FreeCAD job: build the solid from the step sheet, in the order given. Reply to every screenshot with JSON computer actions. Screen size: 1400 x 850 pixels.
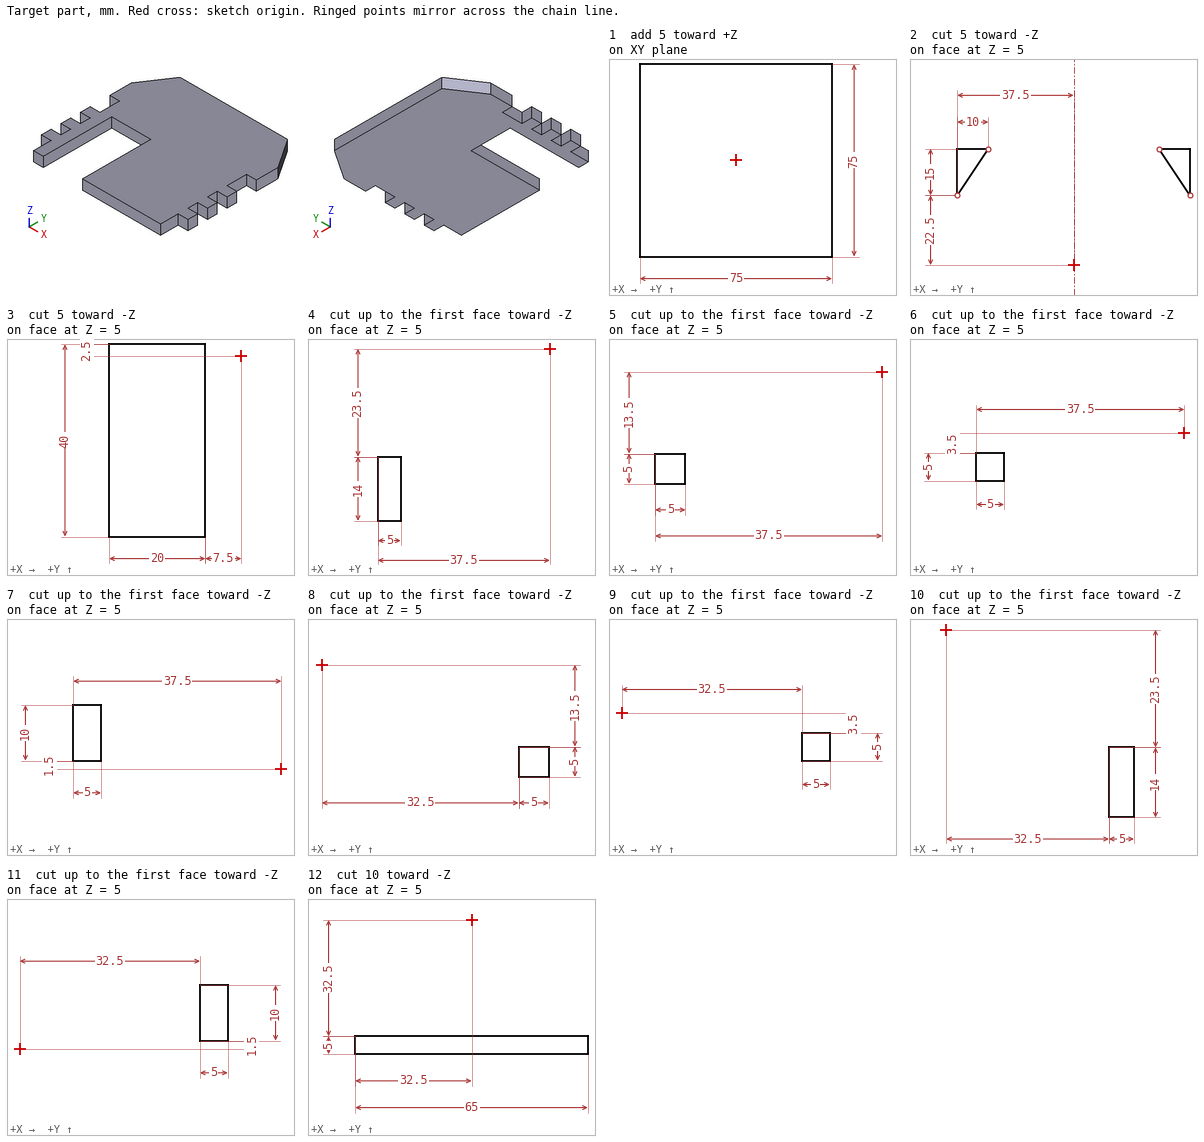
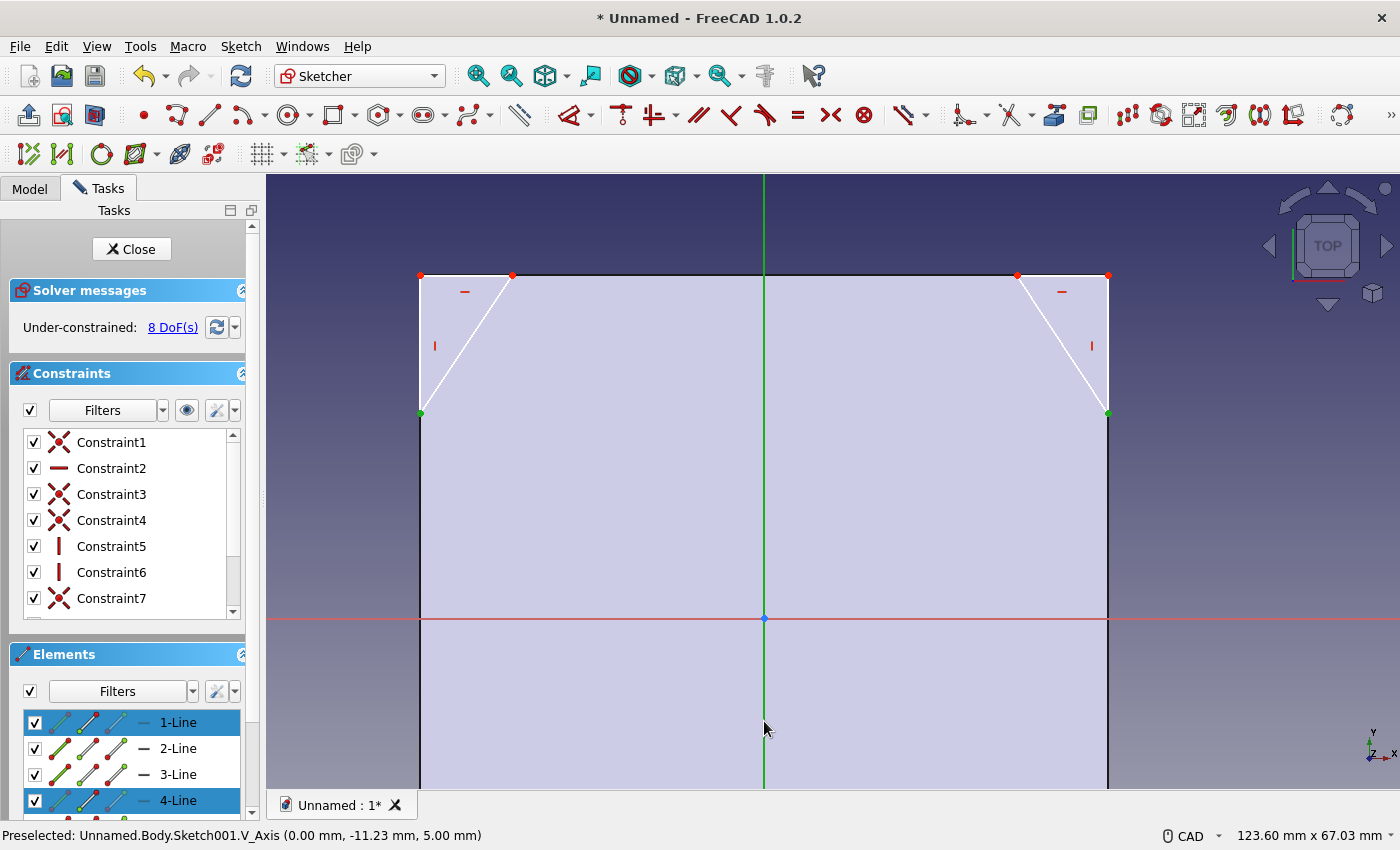
{"action": "left_click", "coordinate": [831, 116]}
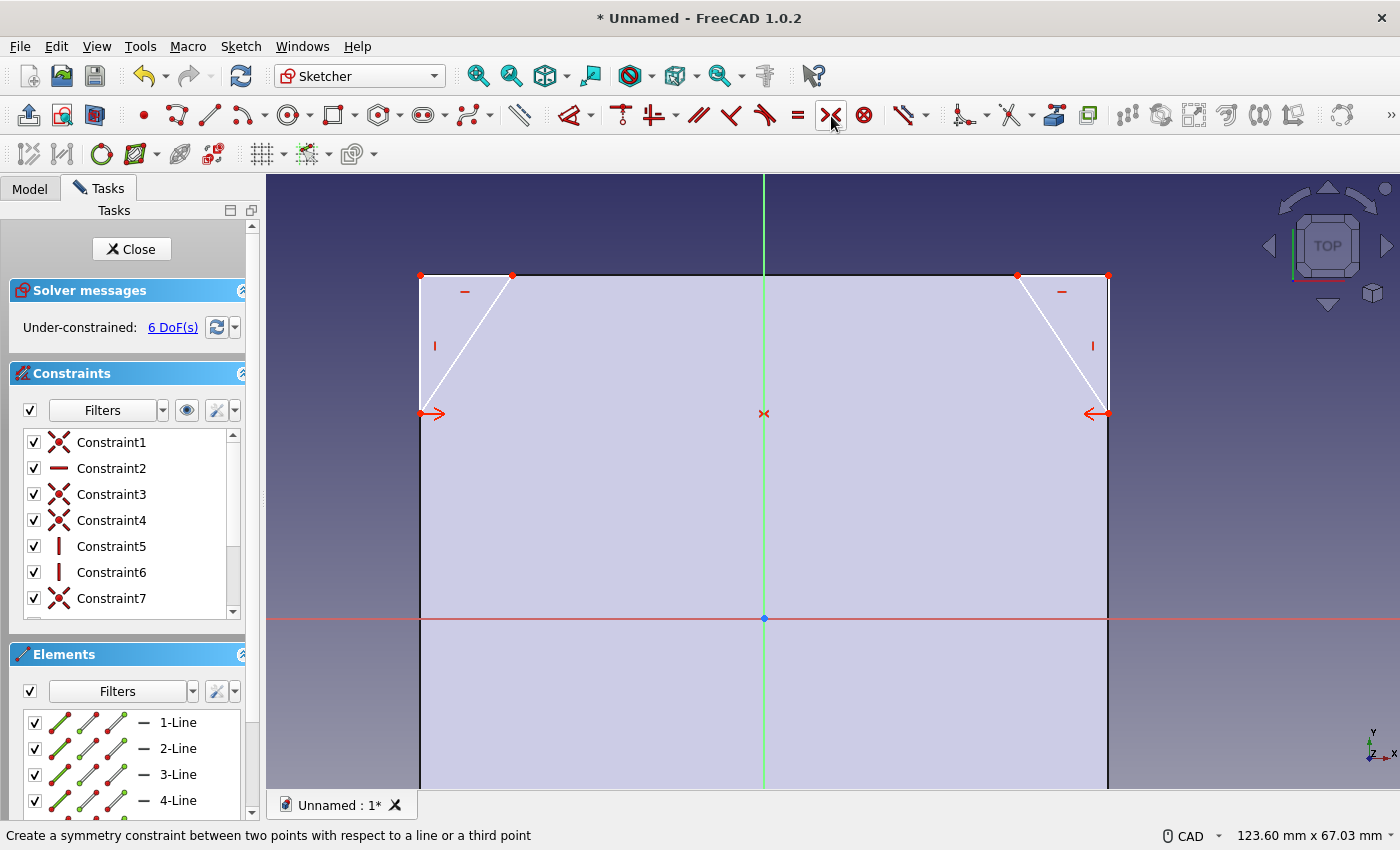
{"action": "left_click", "coordinate": [512, 276]}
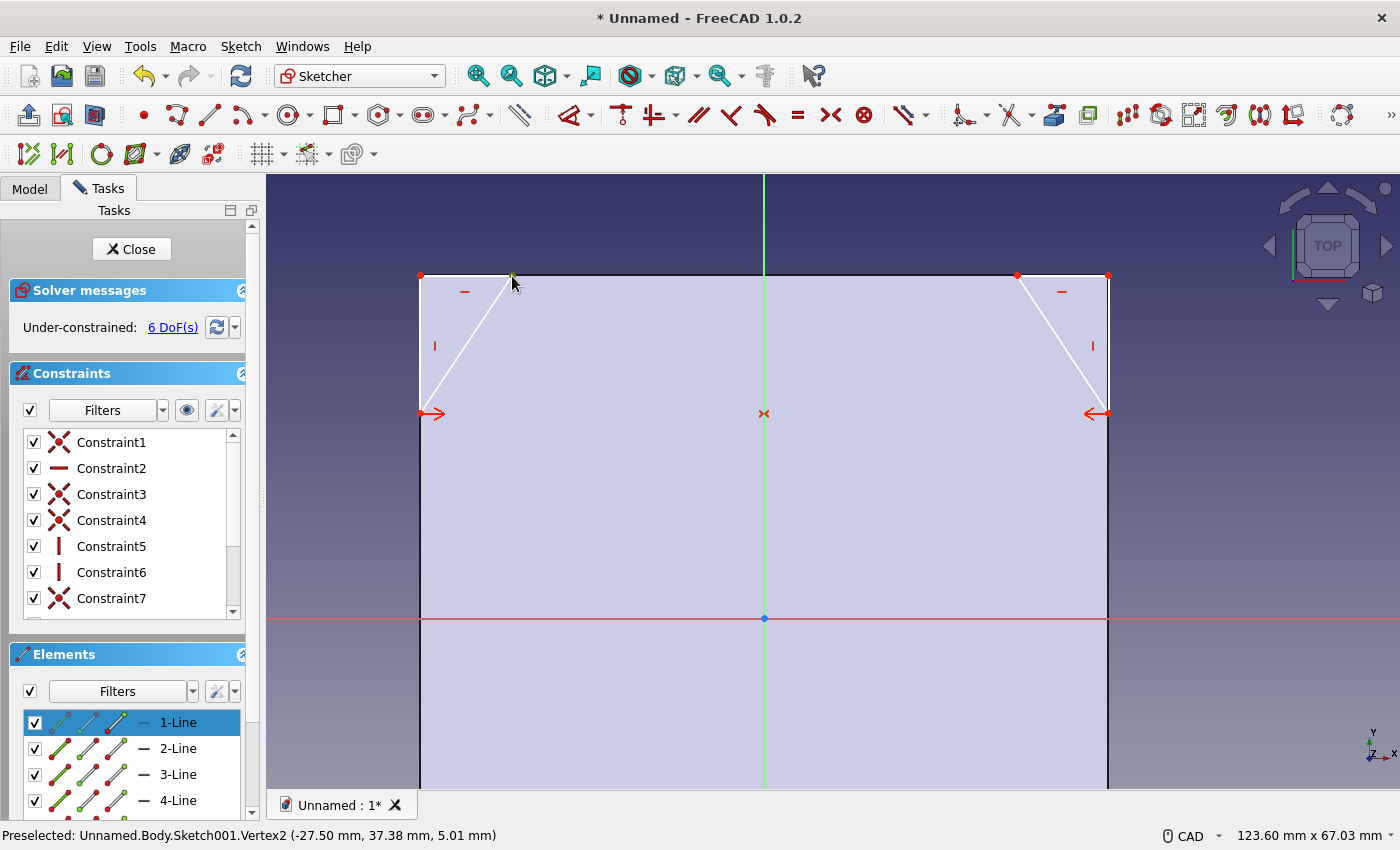
{"action": "left_click", "coordinate": [1017, 276]}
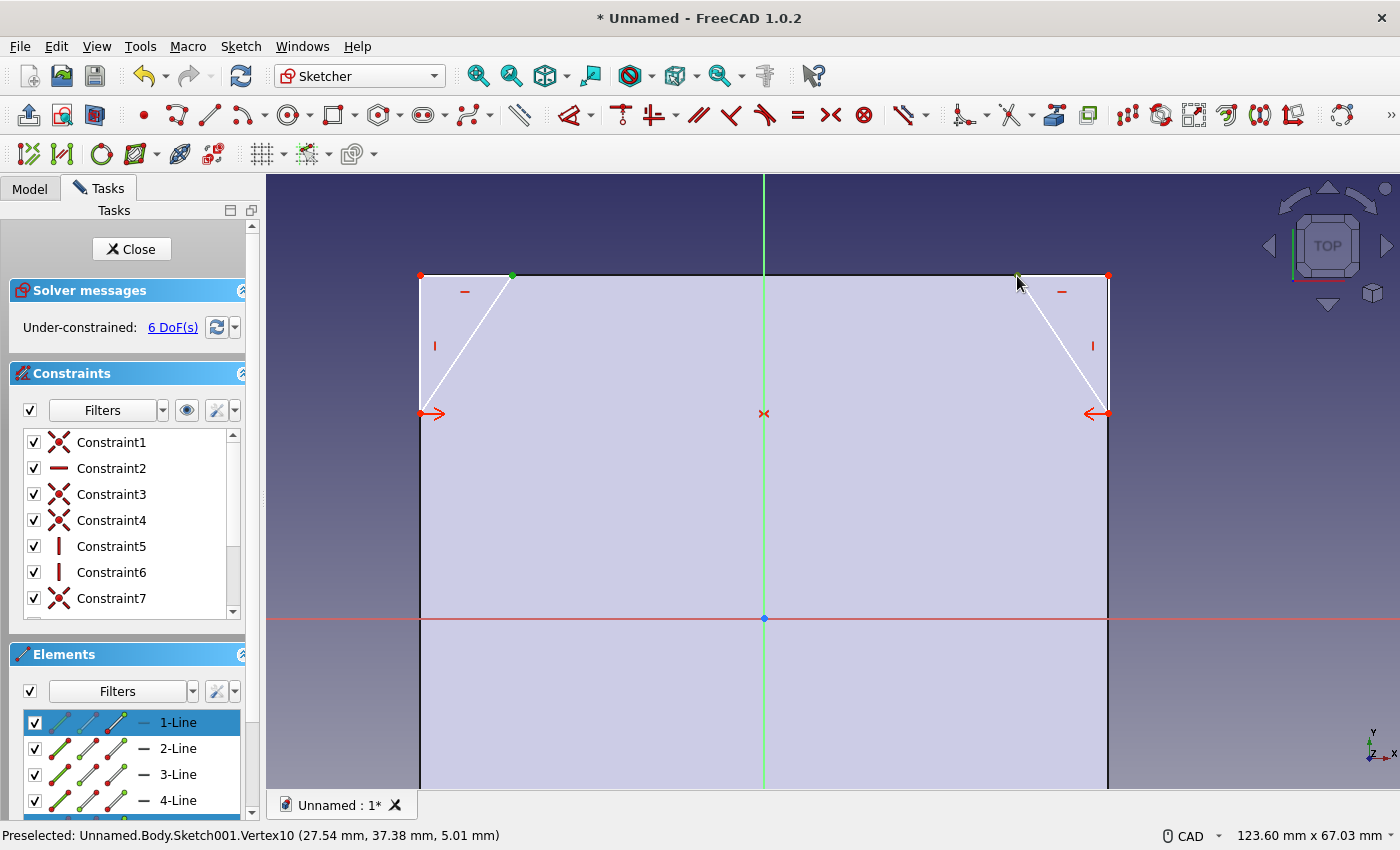
{"action": "left_click", "coordinate": [764, 721]}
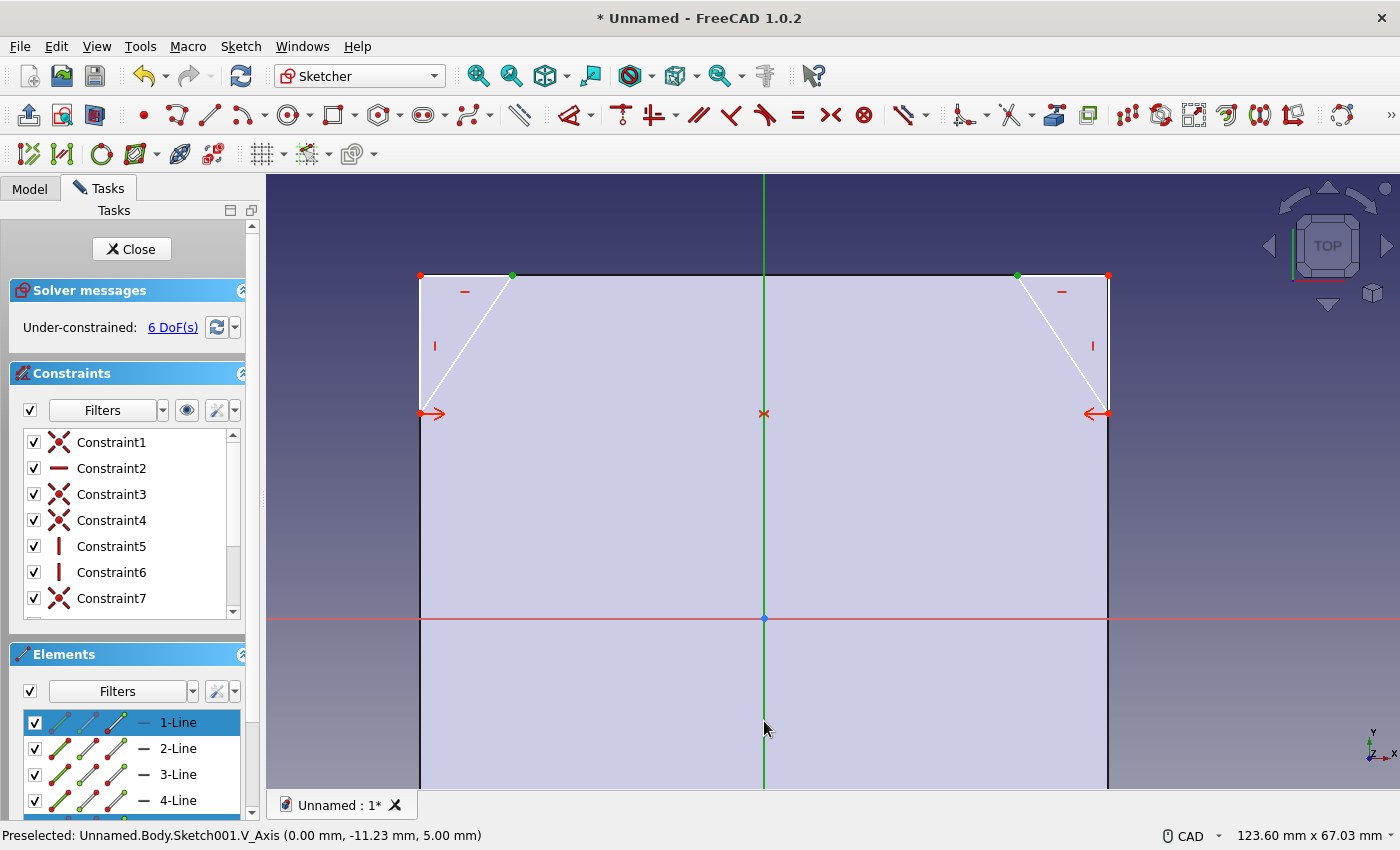
{"action": "left_click", "coordinate": [831, 116]}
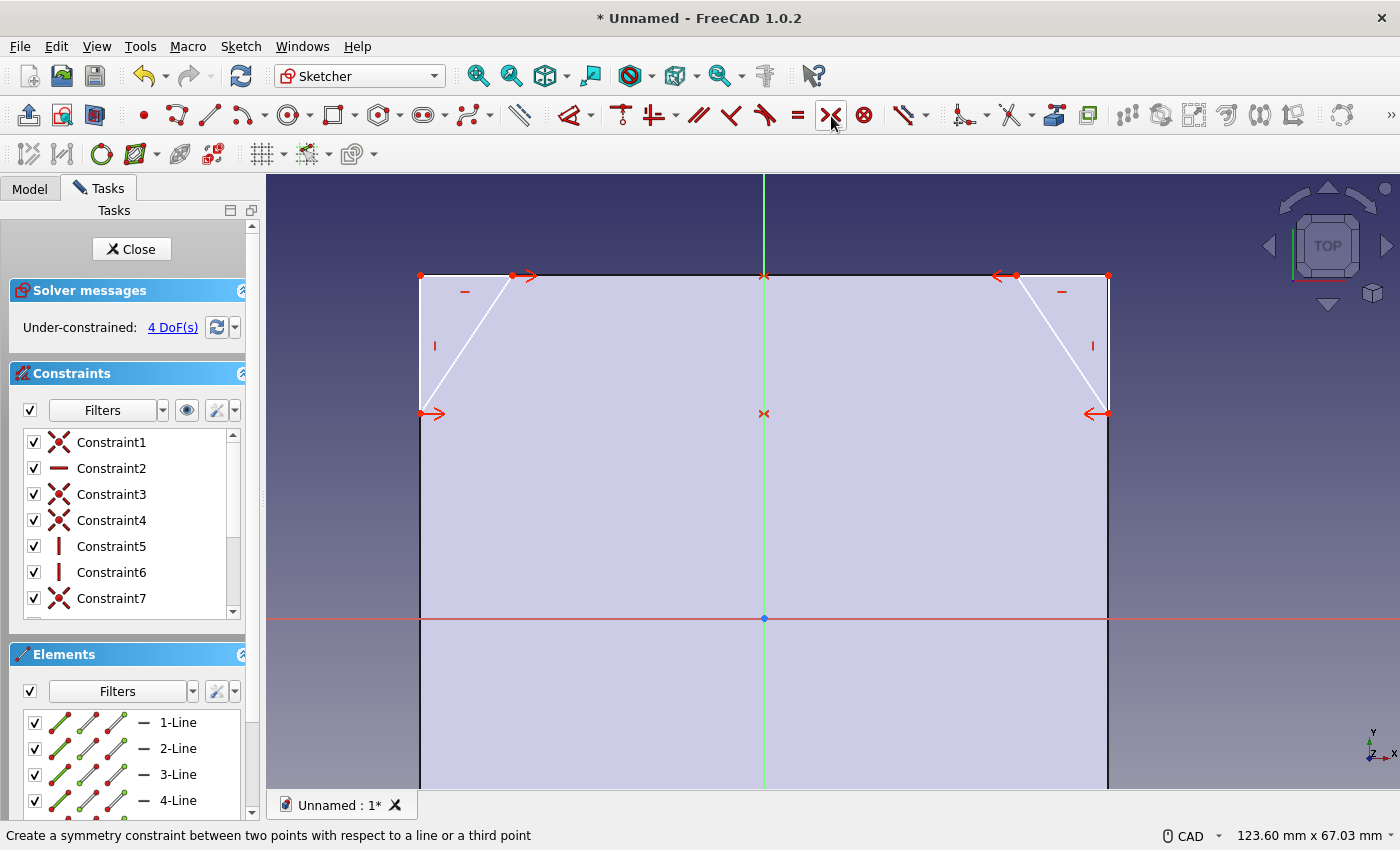
{"action": "left_click", "coordinate": [568, 116]}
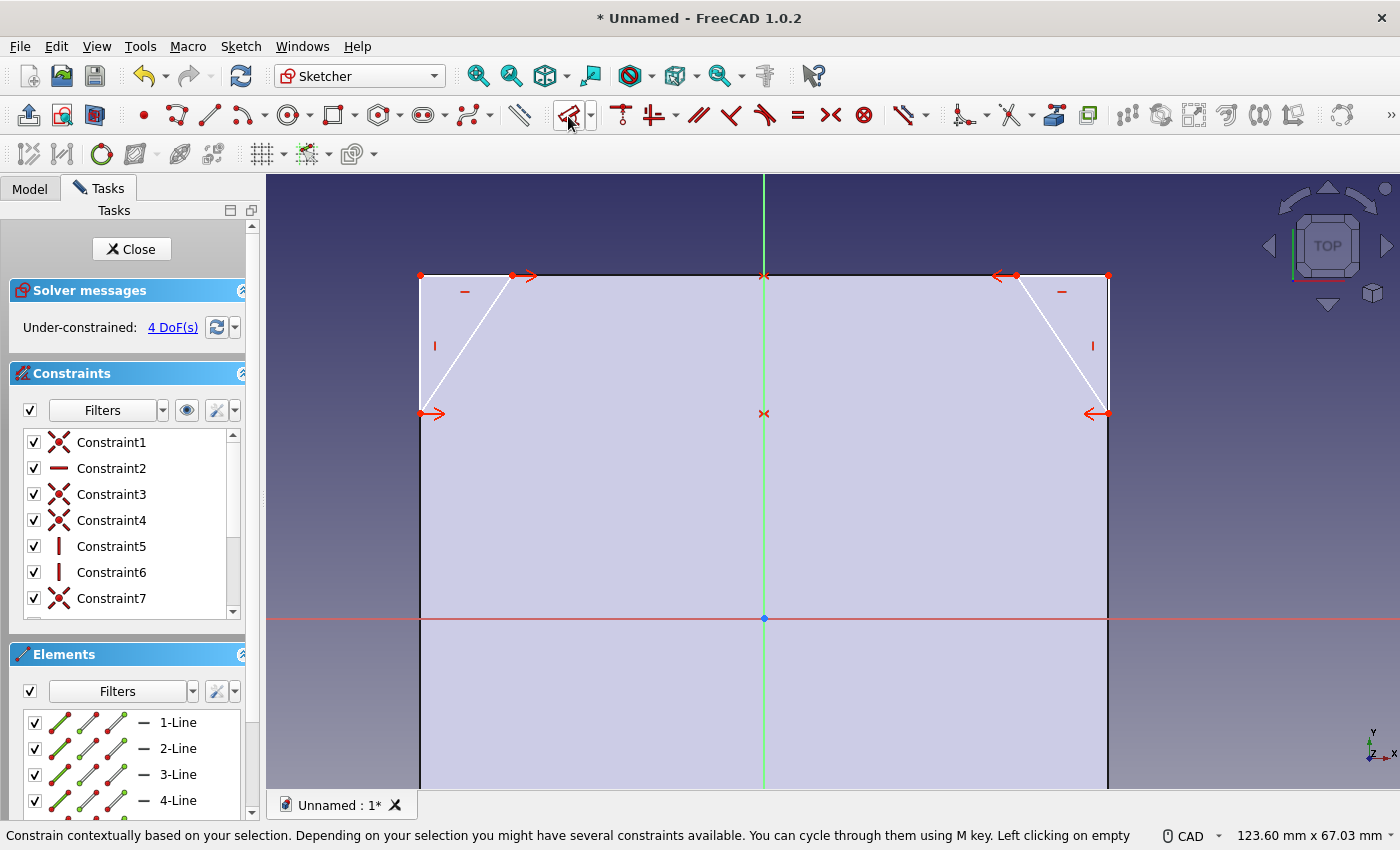
{"action": "left_click", "coordinate": [484, 276]}
{"action": "left_click", "coordinate": [466, 242]}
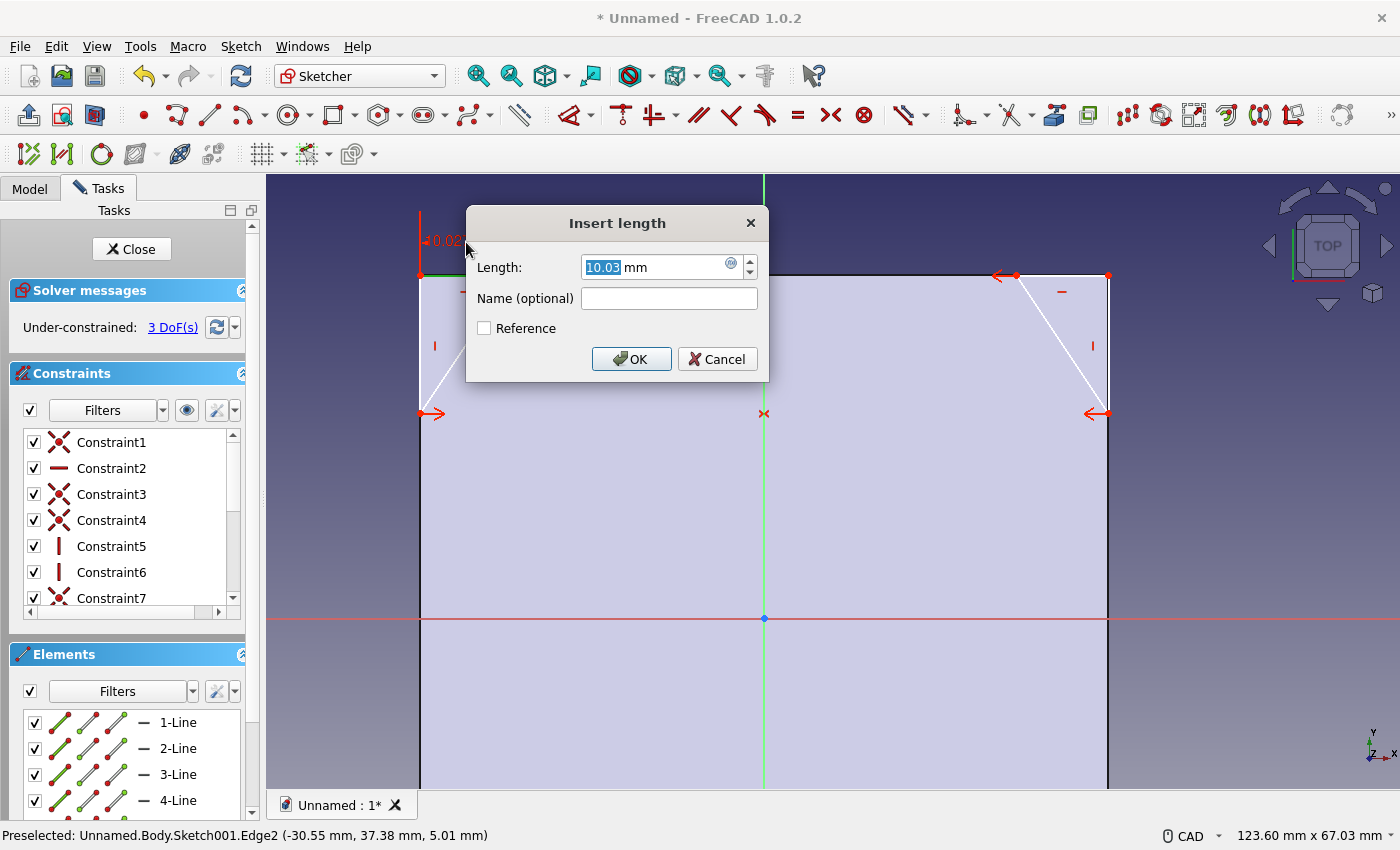
{"action": "type", "text": "10"}
{"action": "key", "text": "Return"}